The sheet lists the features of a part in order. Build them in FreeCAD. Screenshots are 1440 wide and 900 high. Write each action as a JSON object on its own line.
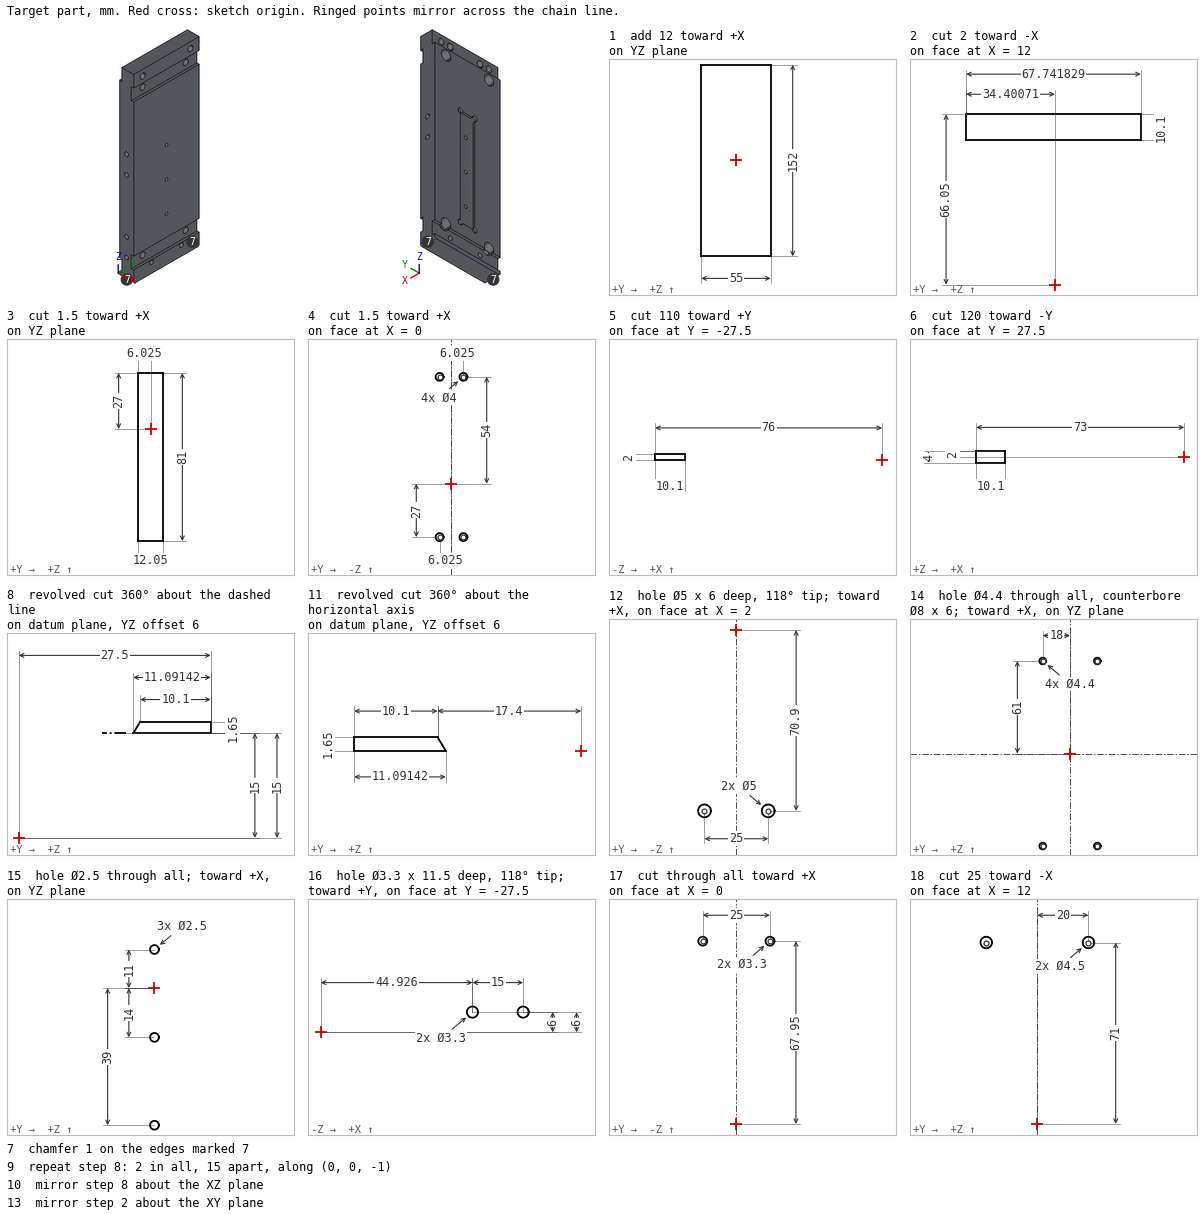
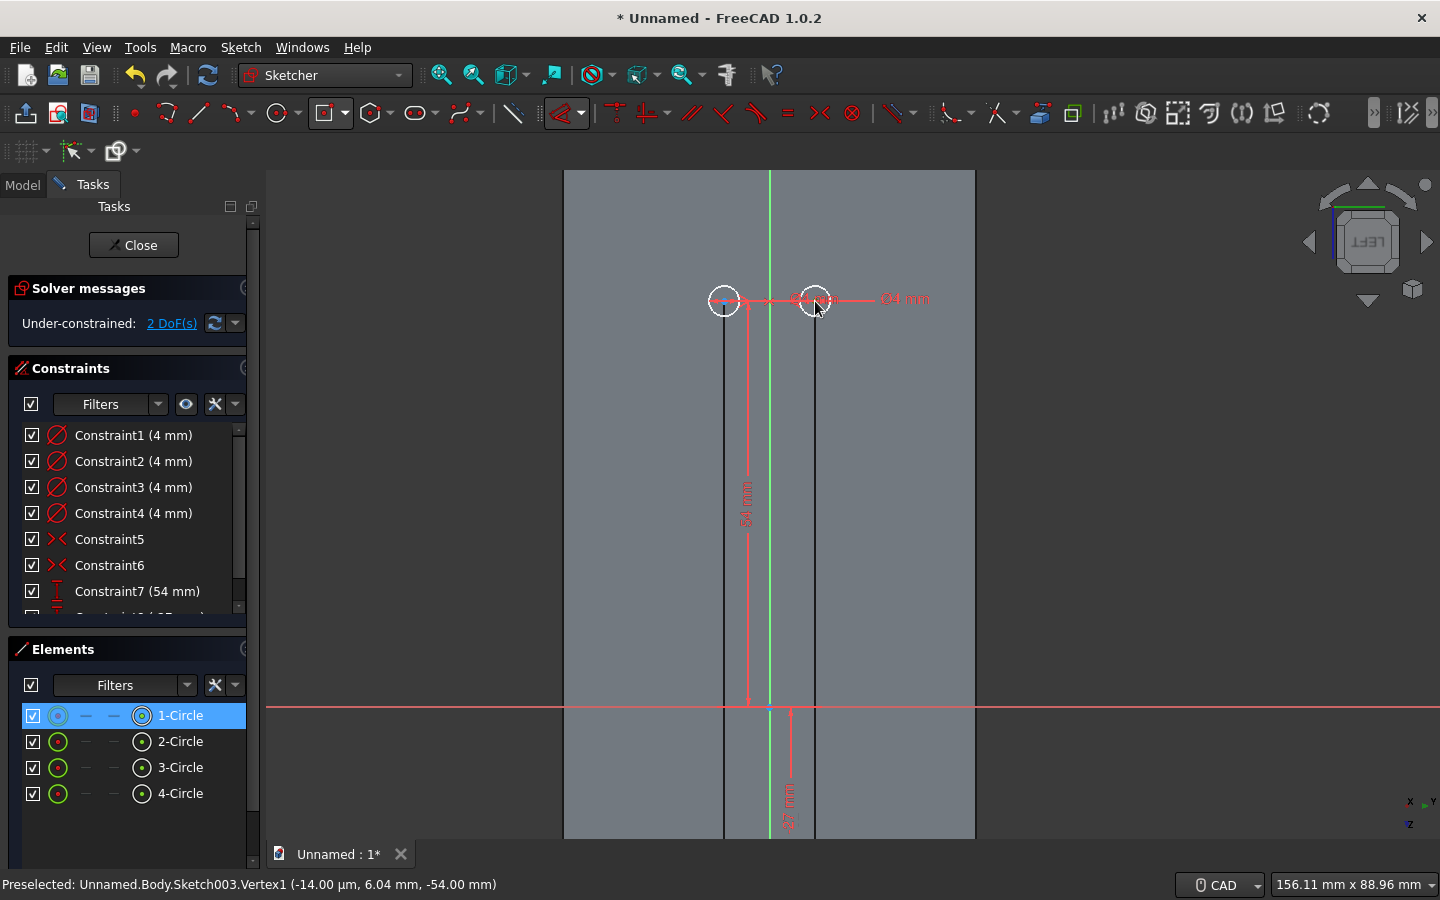
{"action": "left_click", "coordinate": [584, 114]}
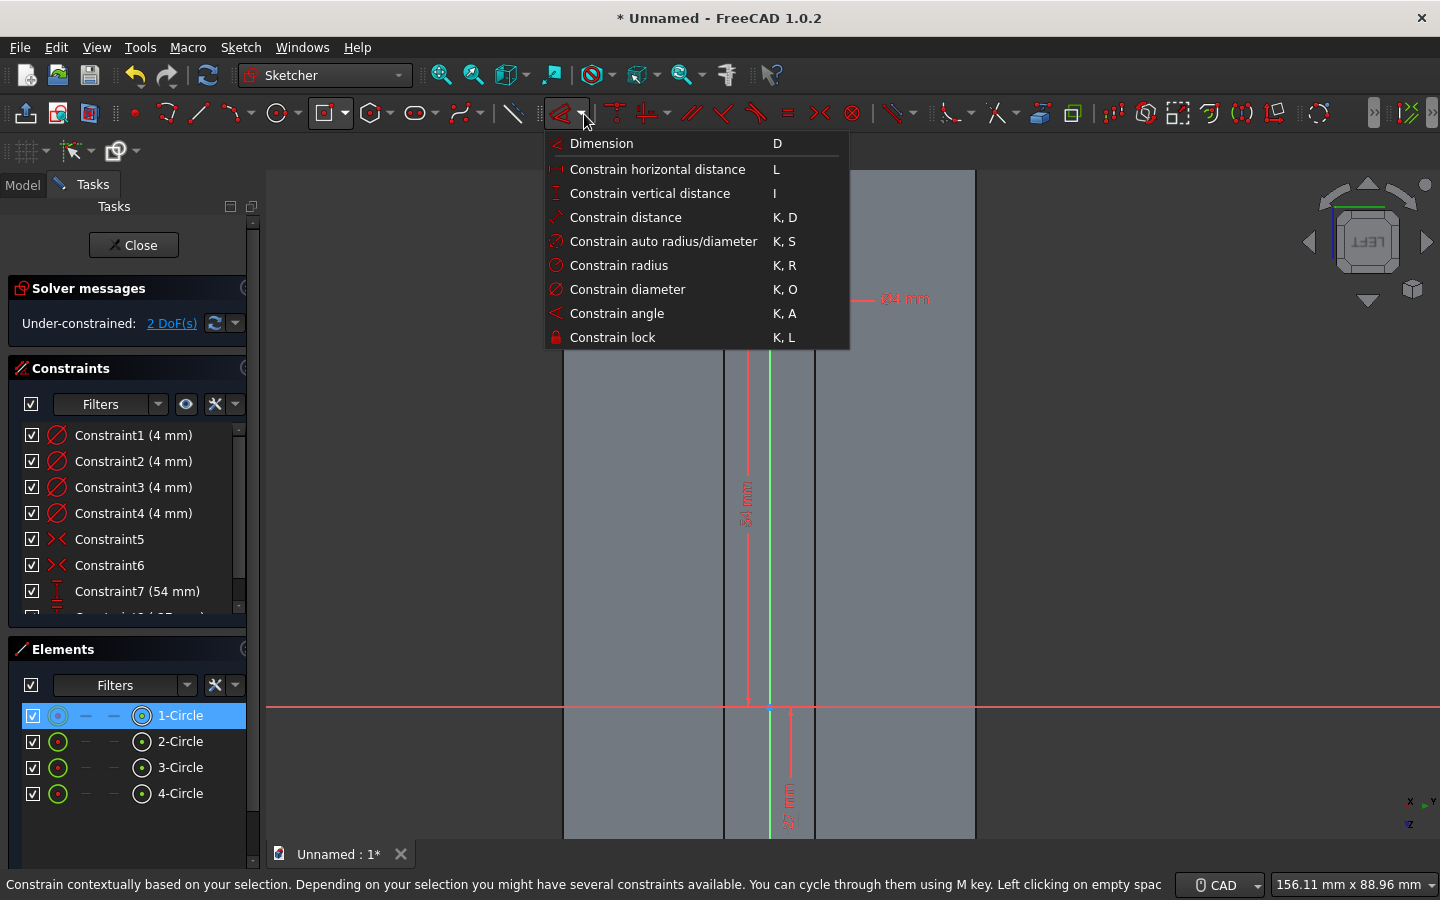
{"action": "left_click", "coordinate": [697, 169]}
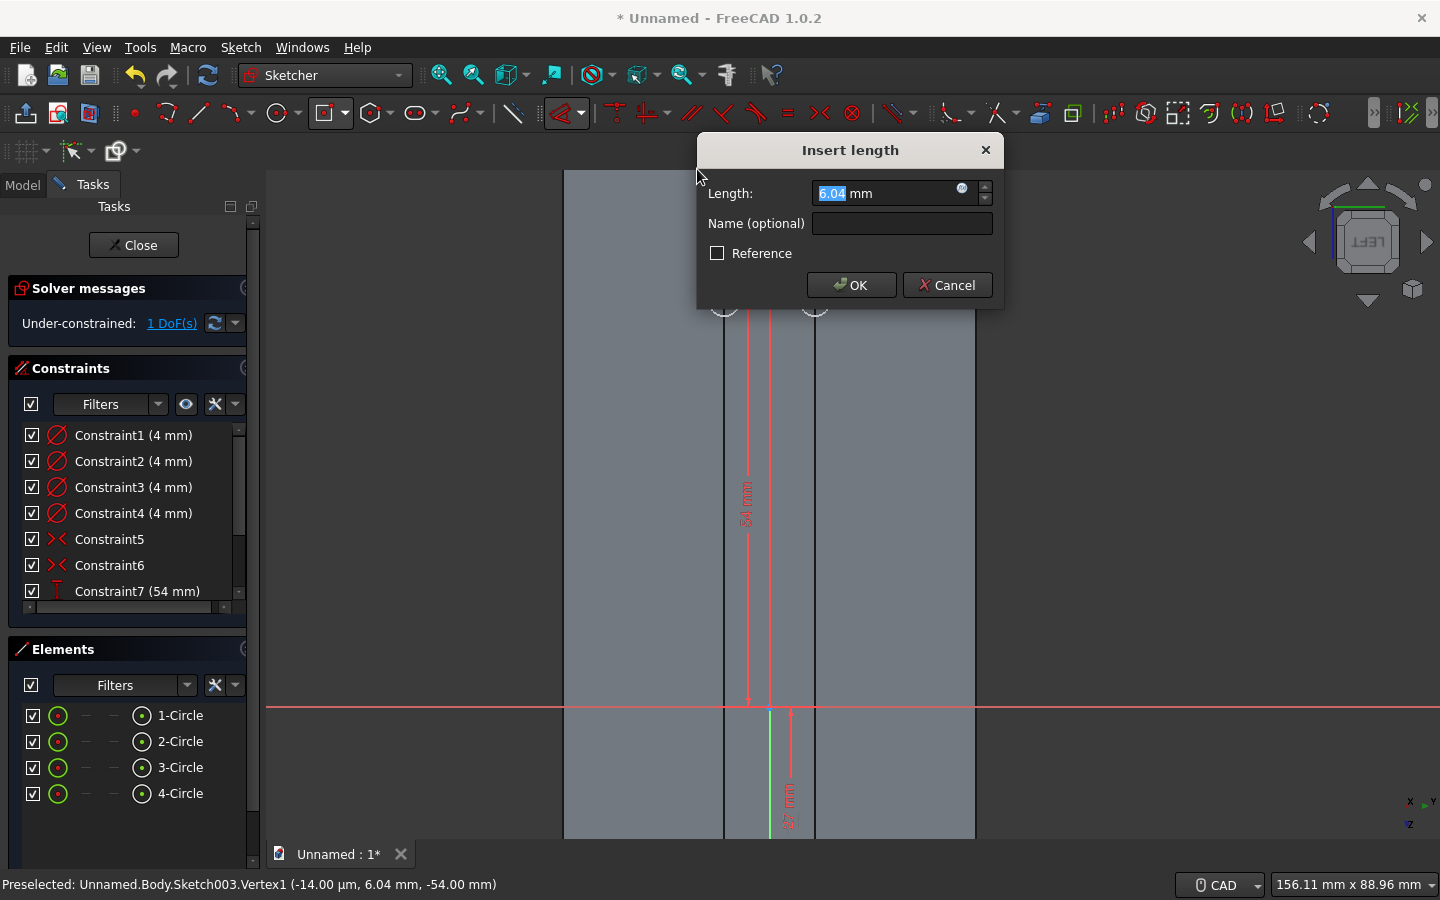
{"action": "type", "text": "6.025"}
{"action": "key", "text": "Return"}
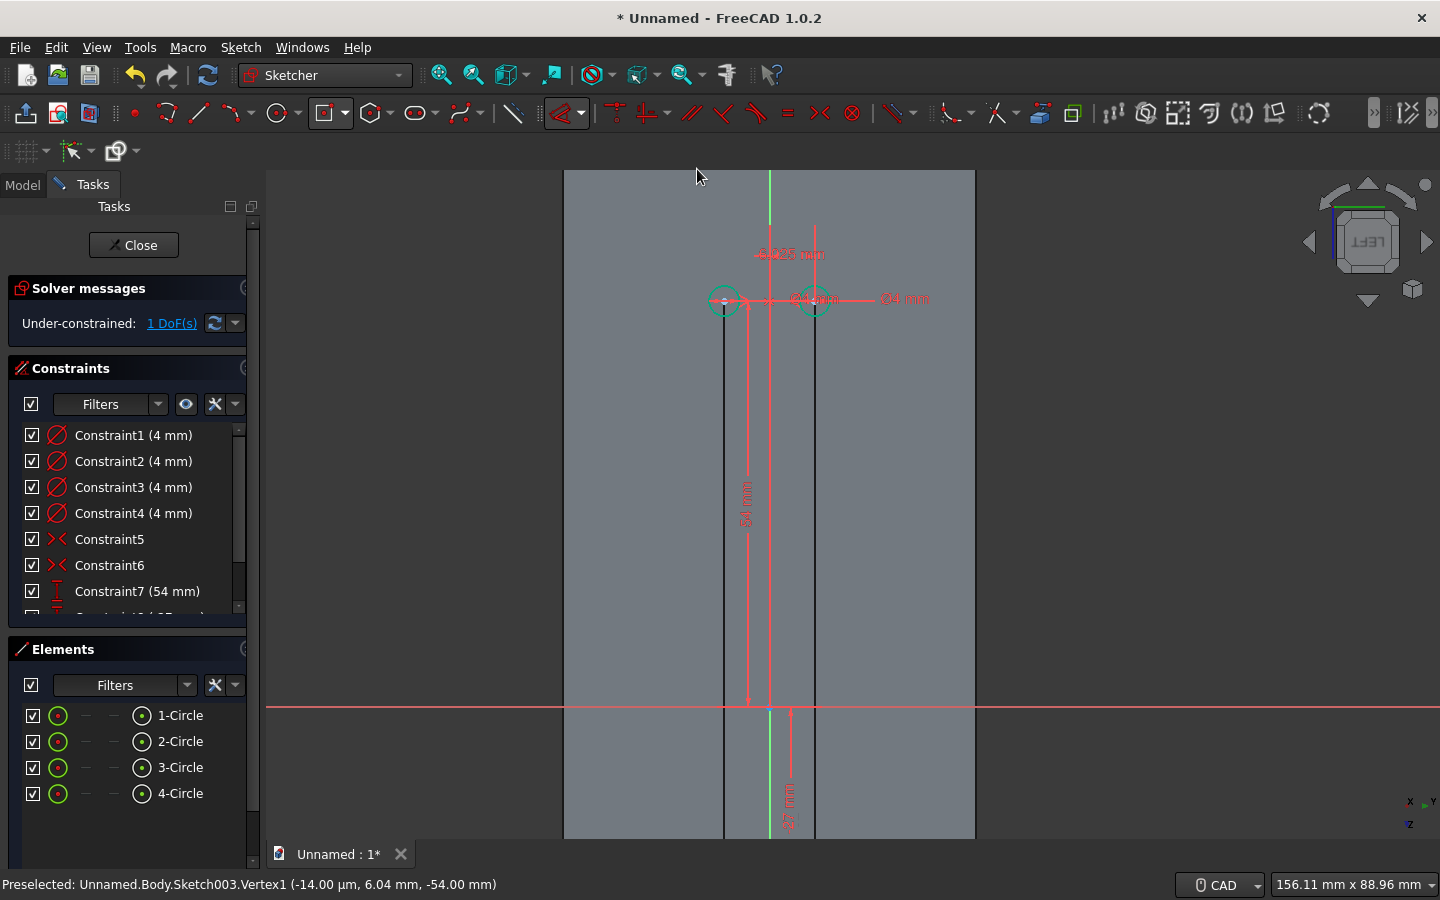
{"action": "scroll", "coordinate": [815, 299], "scroll_direction": "down", "scroll_amount": 2}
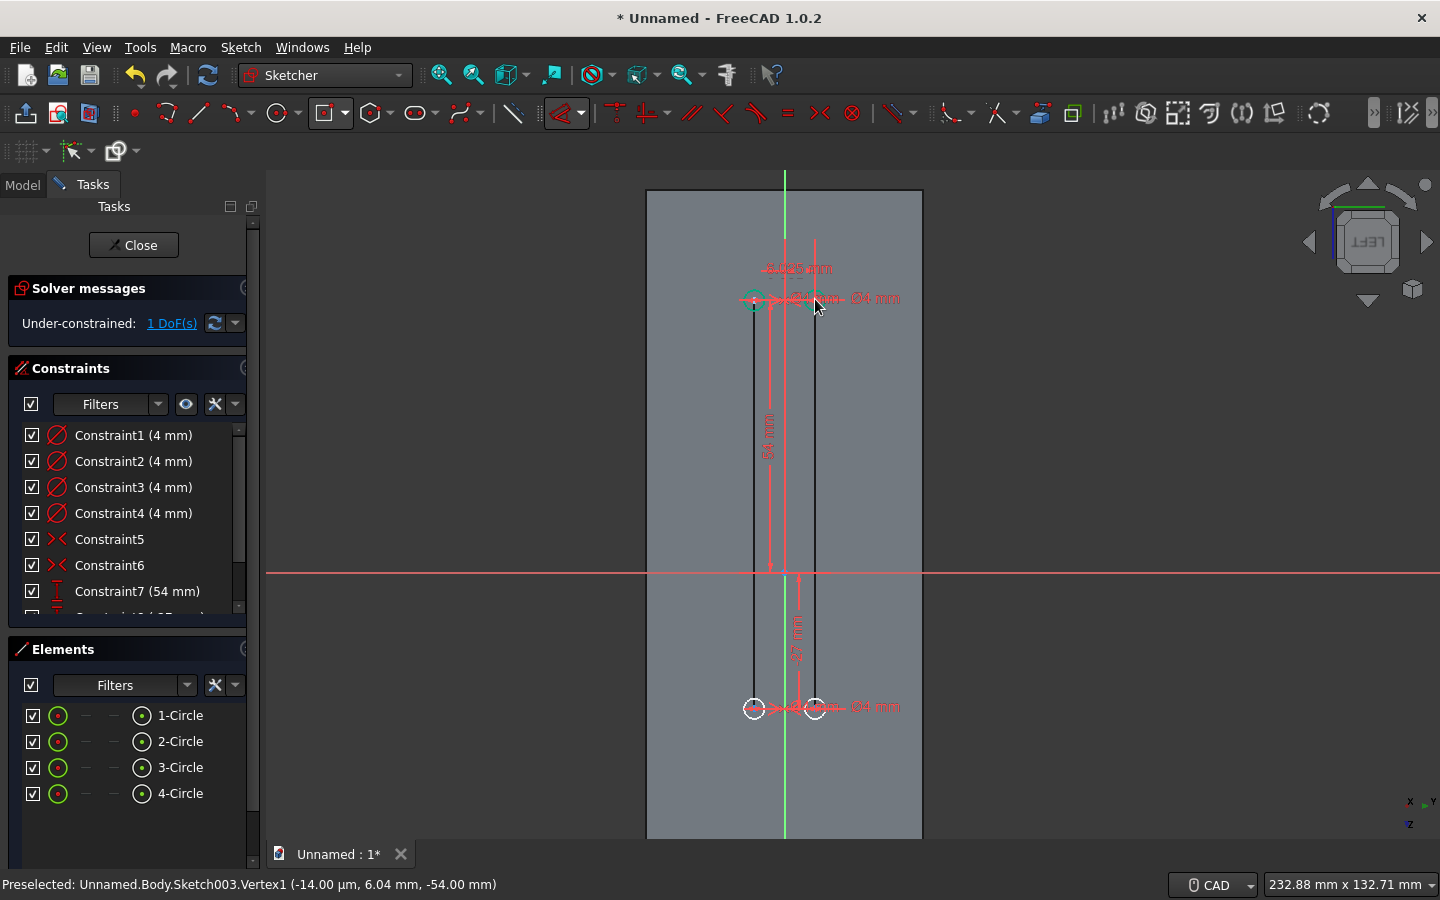
{"action": "scroll", "coordinate": [754, 709], "scroll_direction": "up", "scroll_amount": 2}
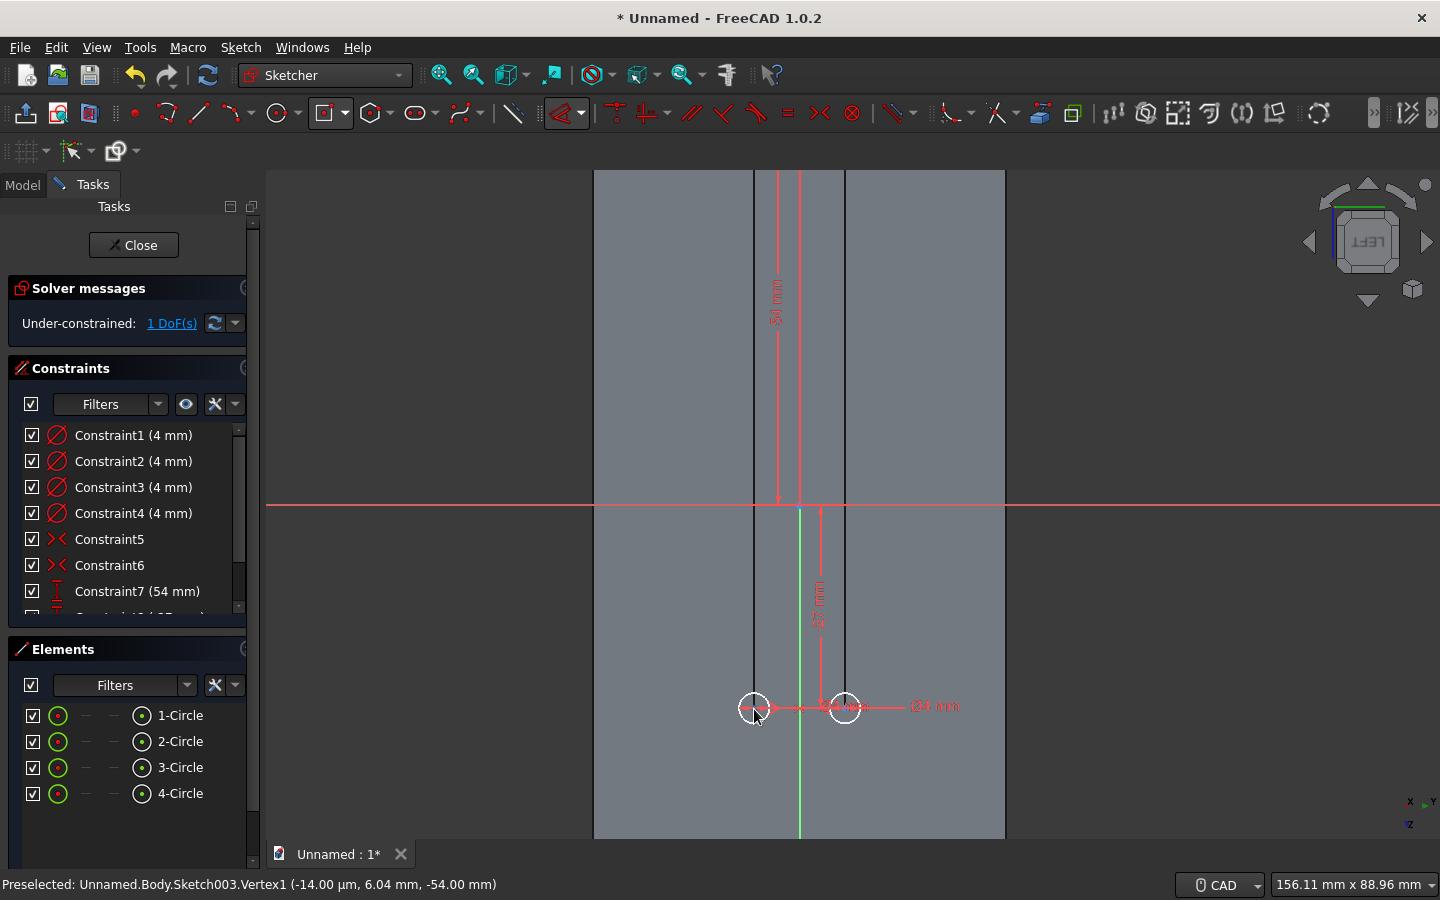
{"action": "left_click", "coordinate": [754, 708]}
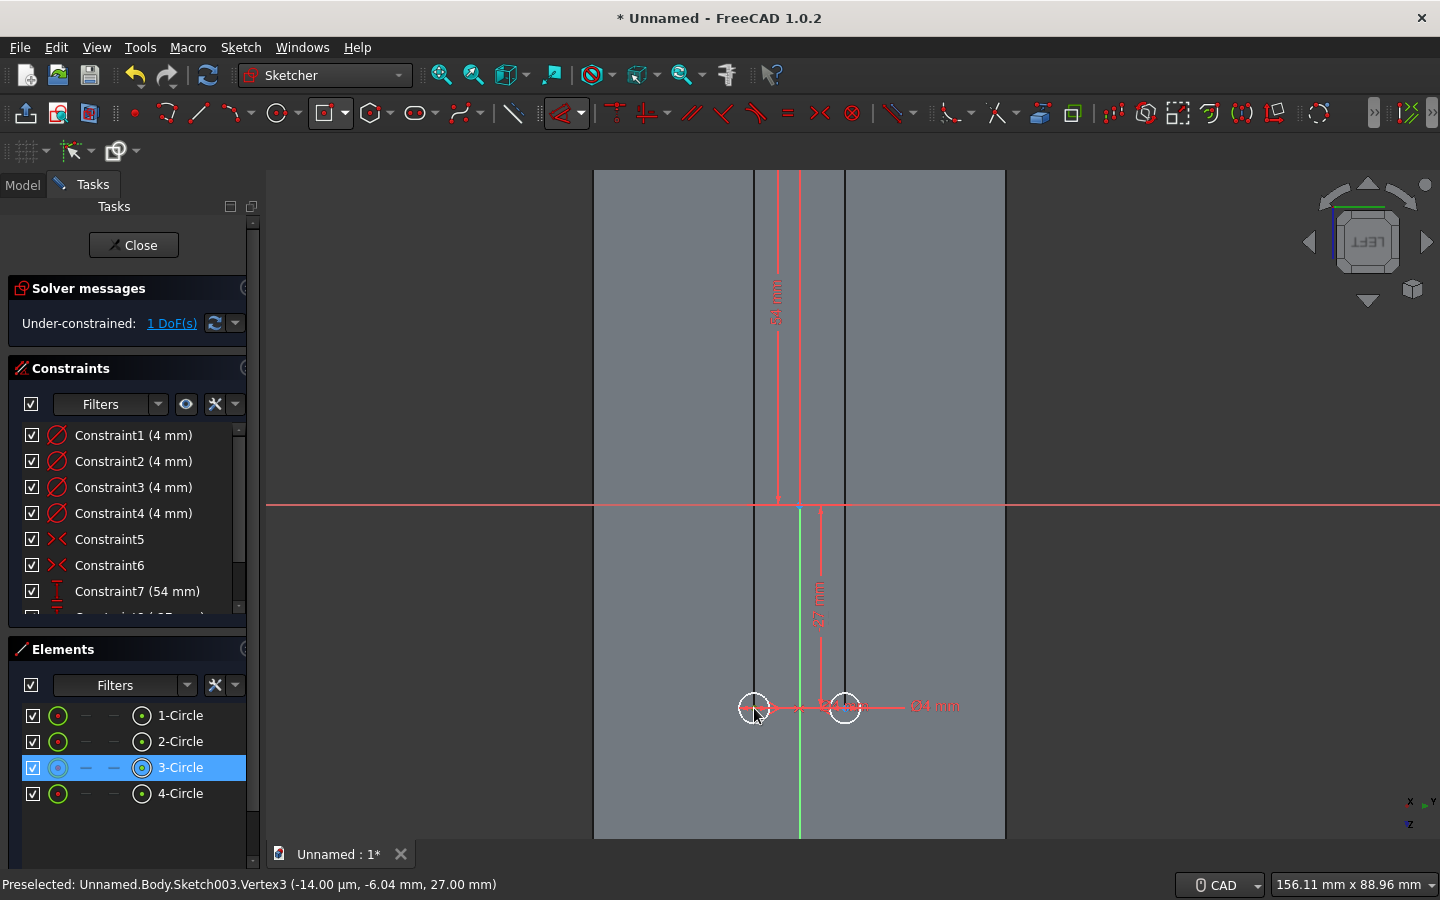
{"action": "left_click", "coordinate": [584, 114]}